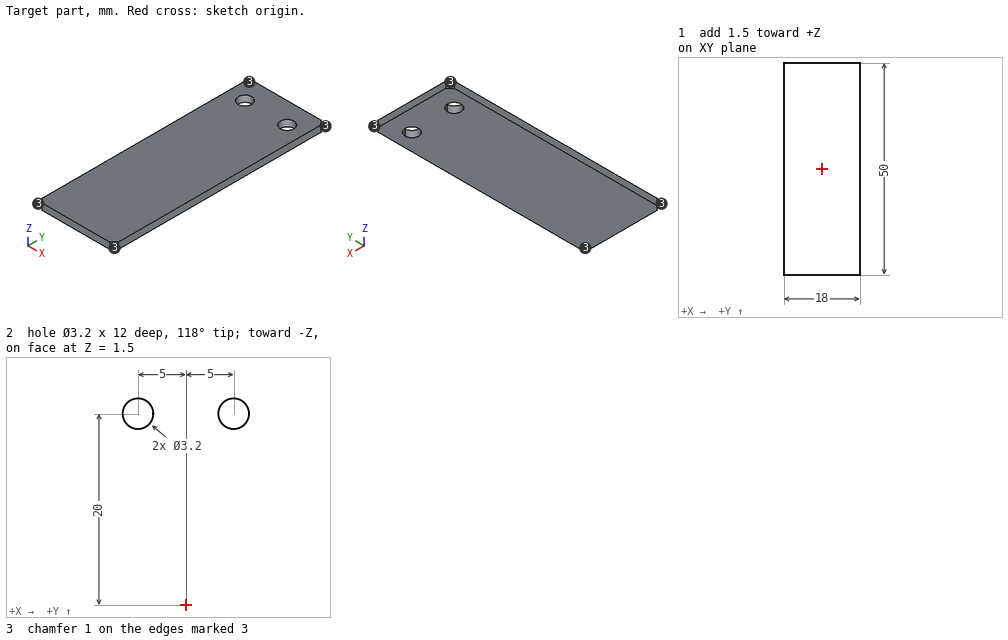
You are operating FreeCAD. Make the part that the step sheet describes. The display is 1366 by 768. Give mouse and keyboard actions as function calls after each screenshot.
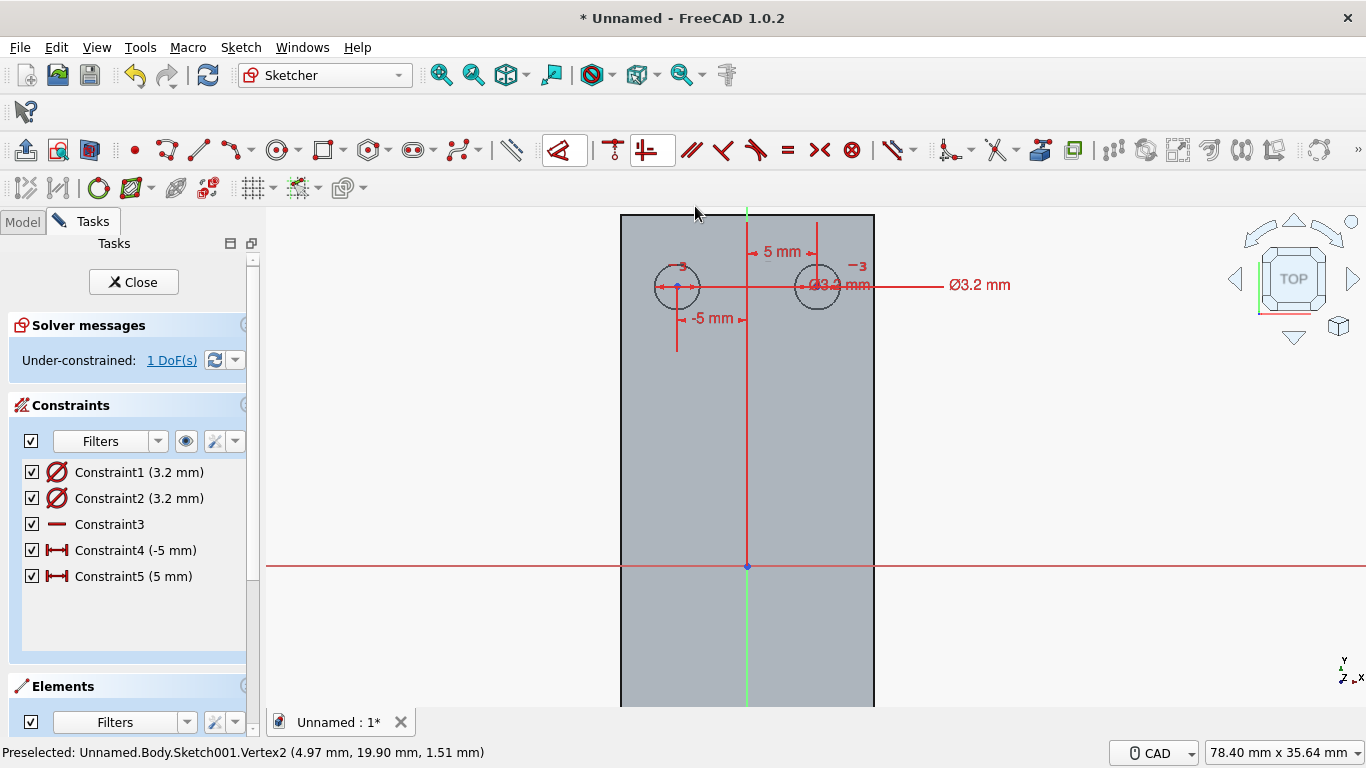
click(677, 287)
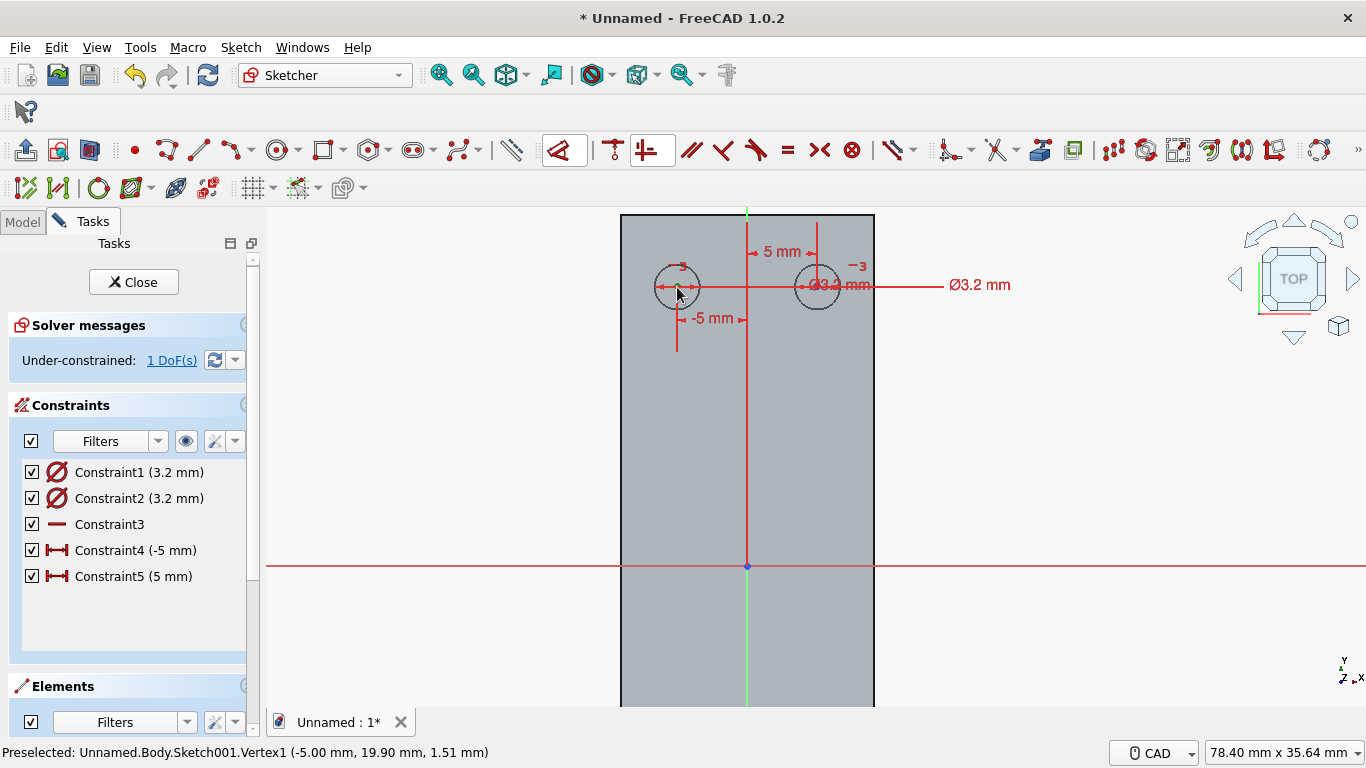
key(i)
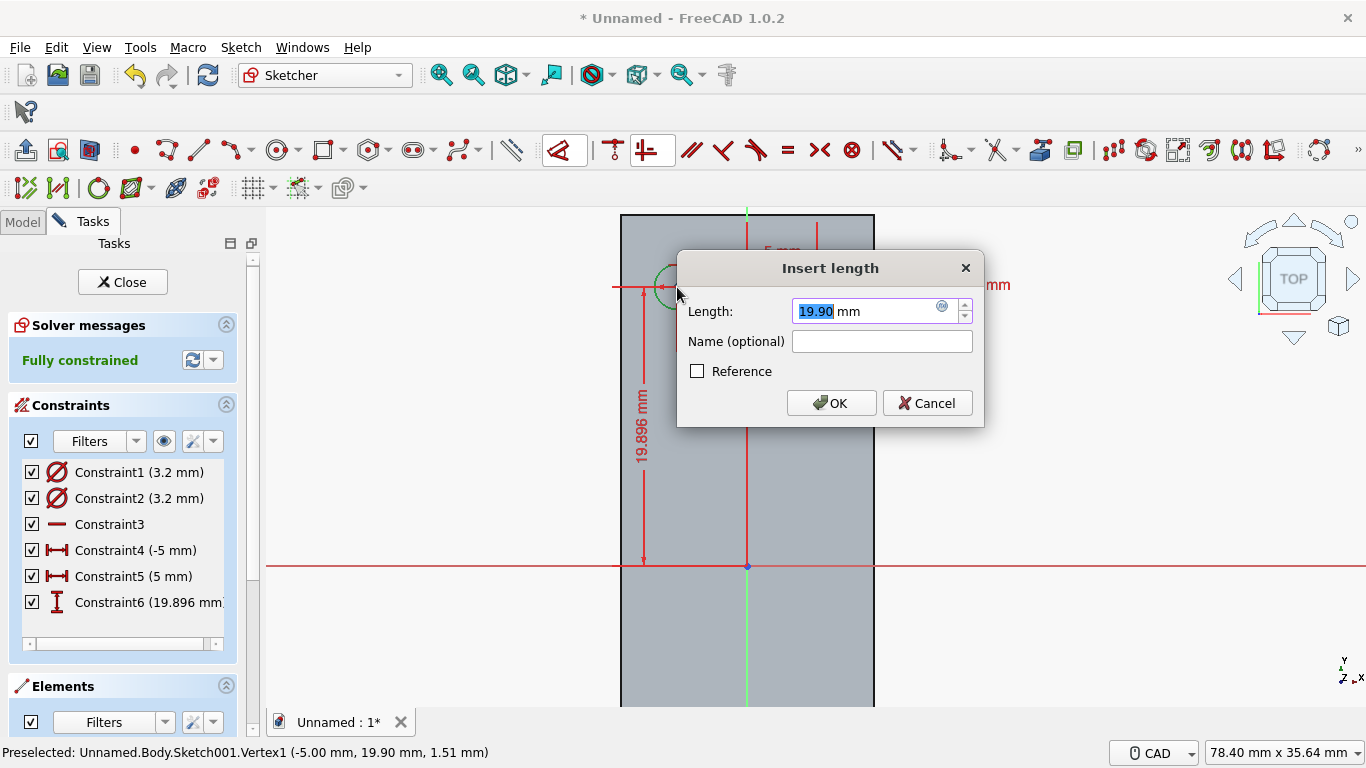
text(20)
key(Return)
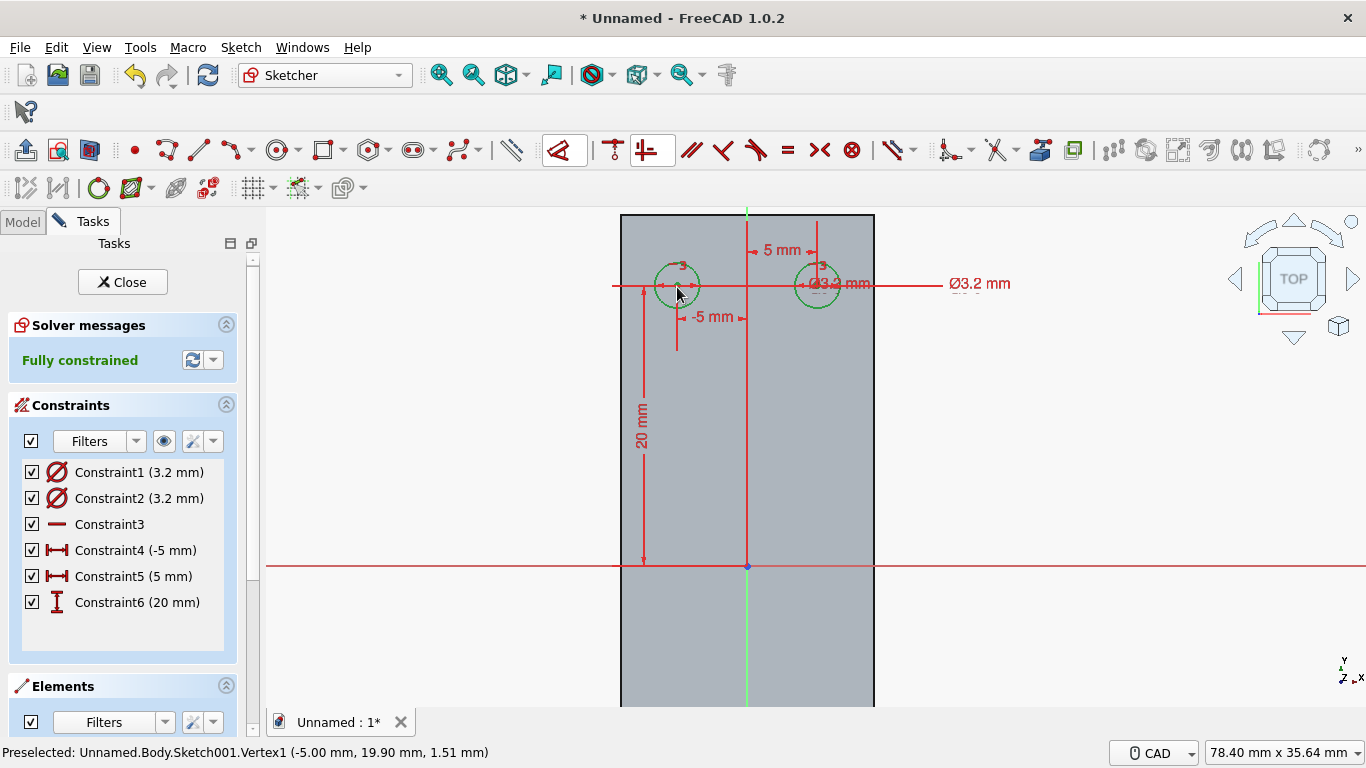
click(123, 282)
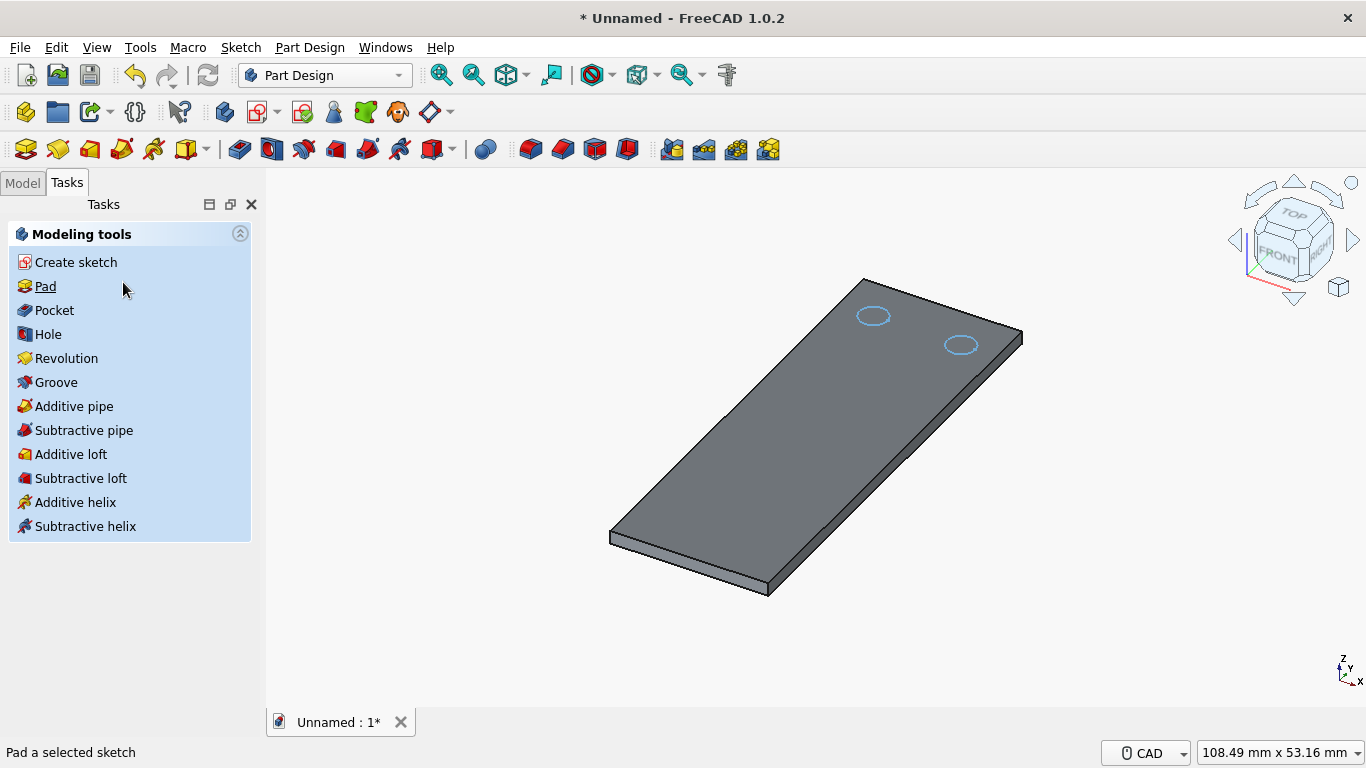
click(272, 150)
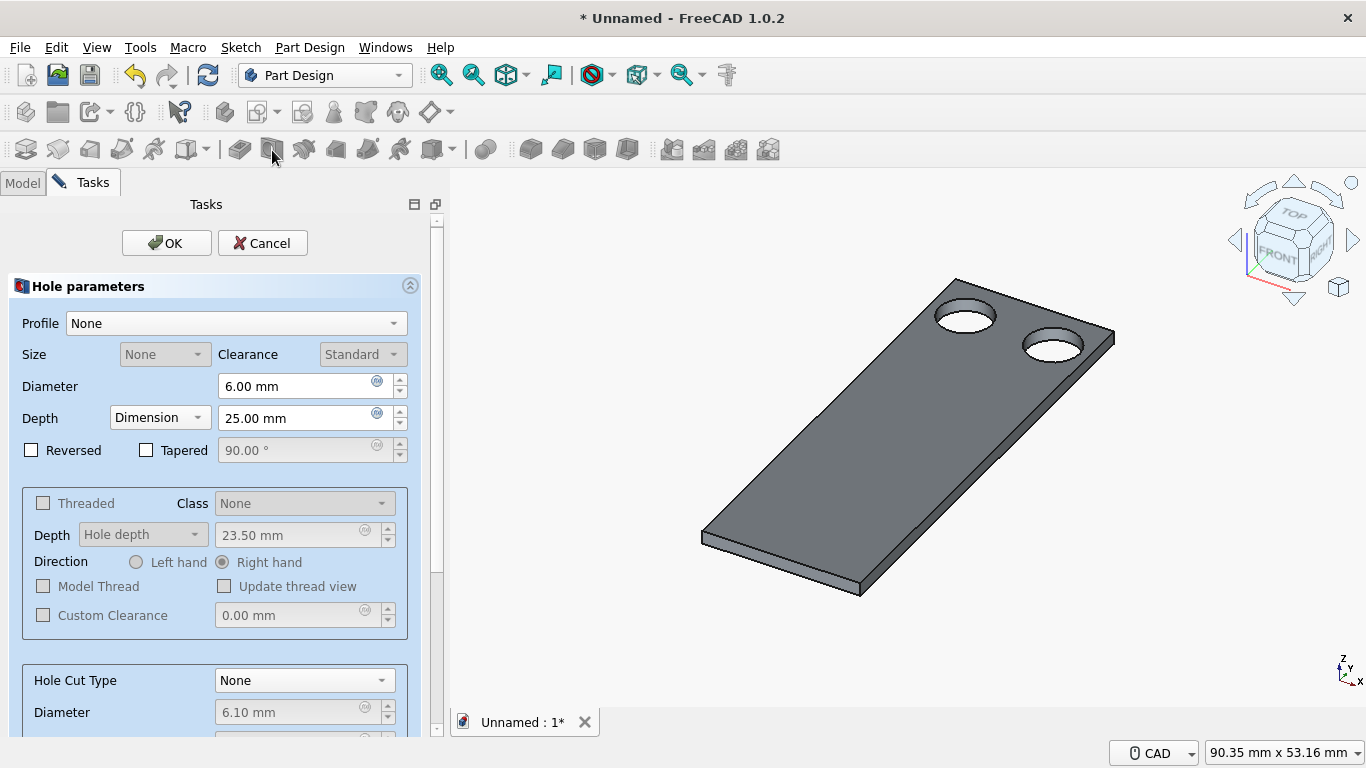
triple_click(305, 386)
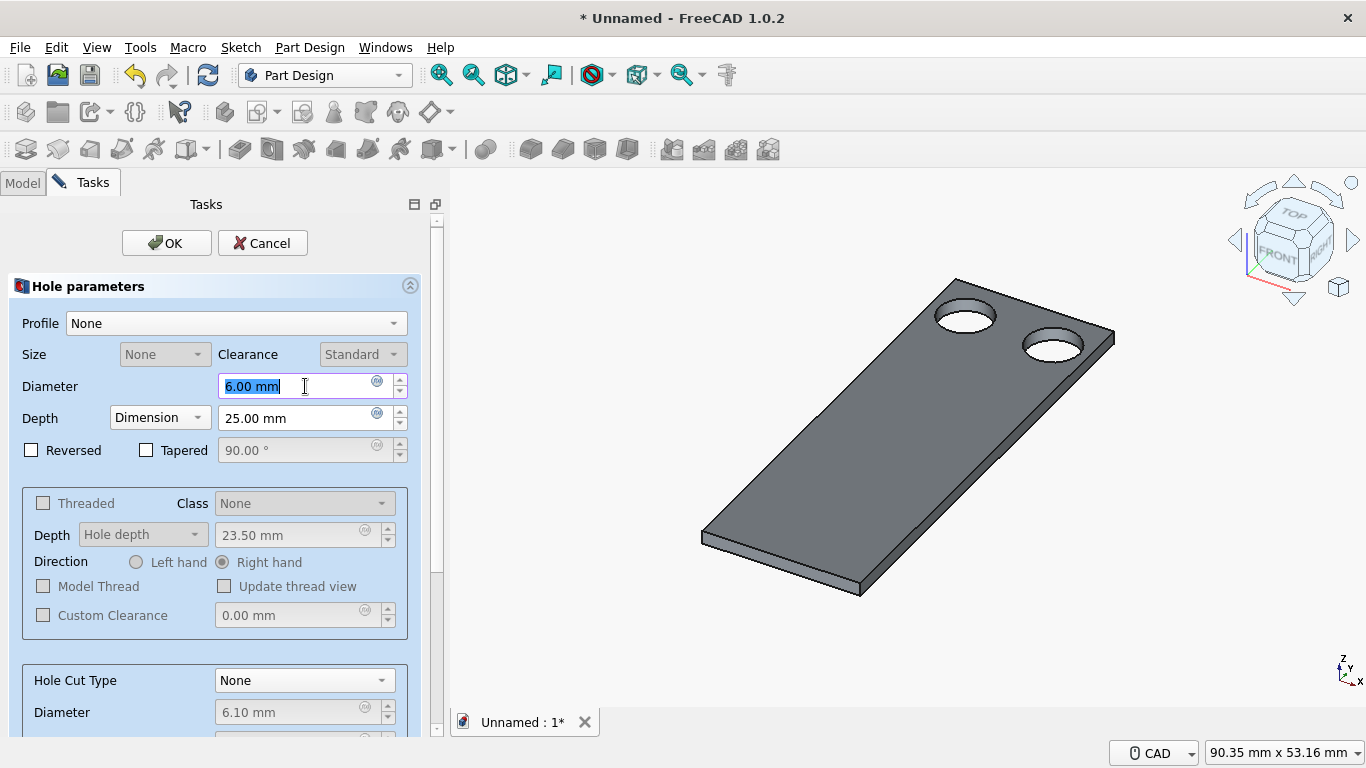
text(3.2)
key(Tab)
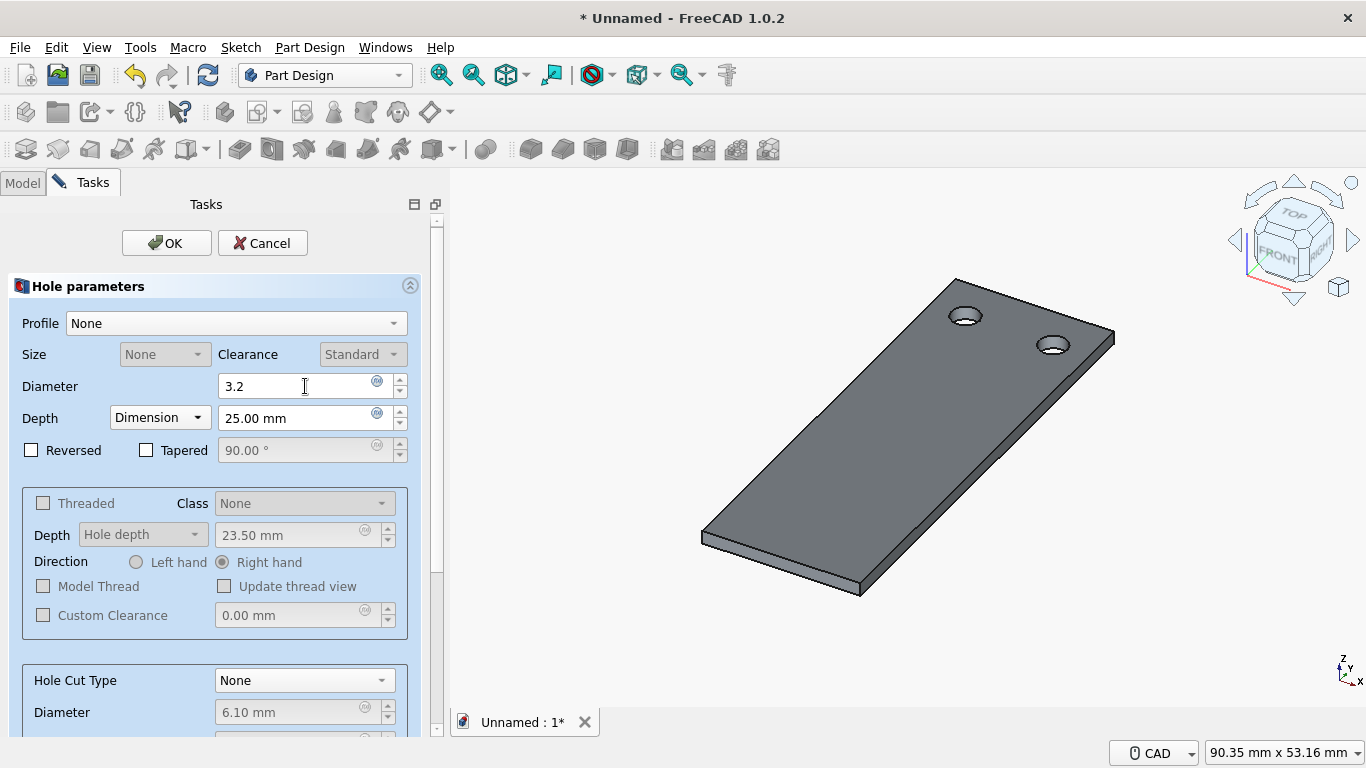
triple_click(305, 418)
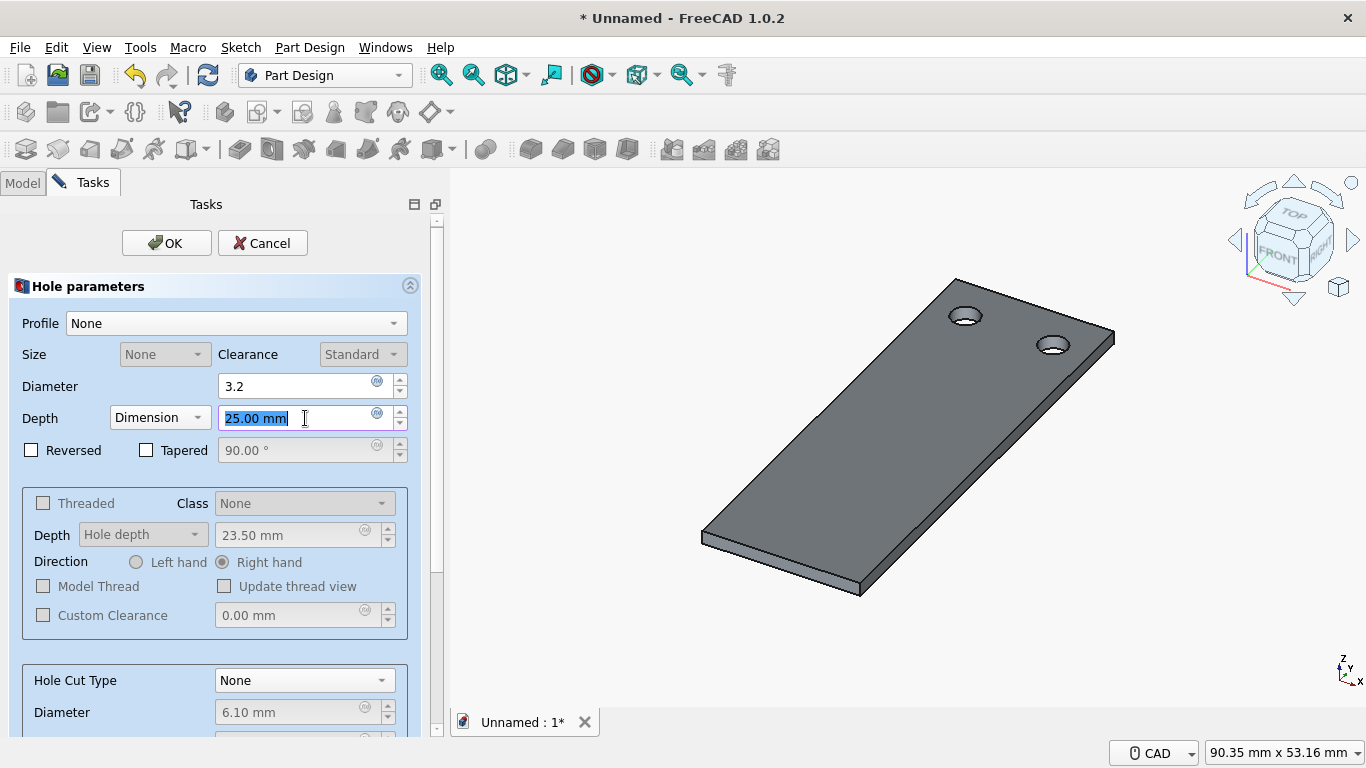
text(12)
key(Tab)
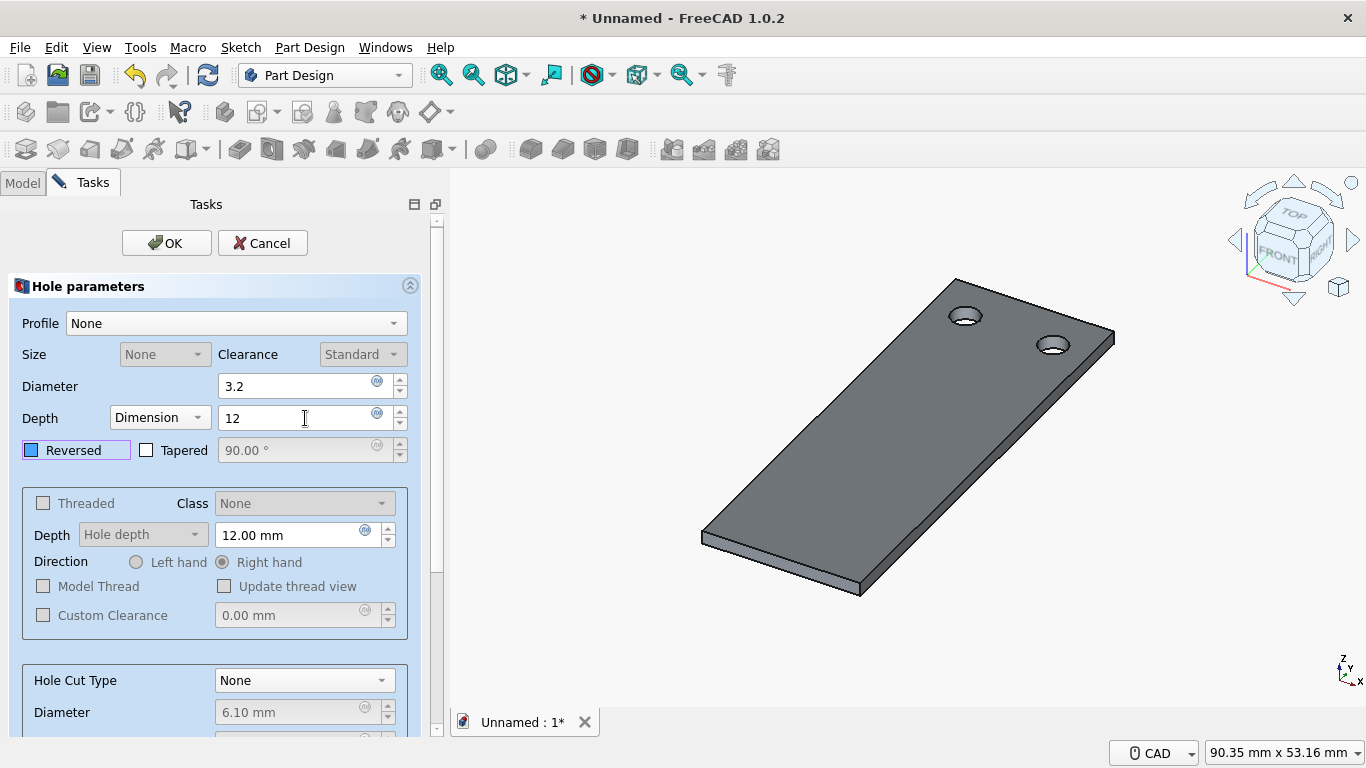
click(167, 243)